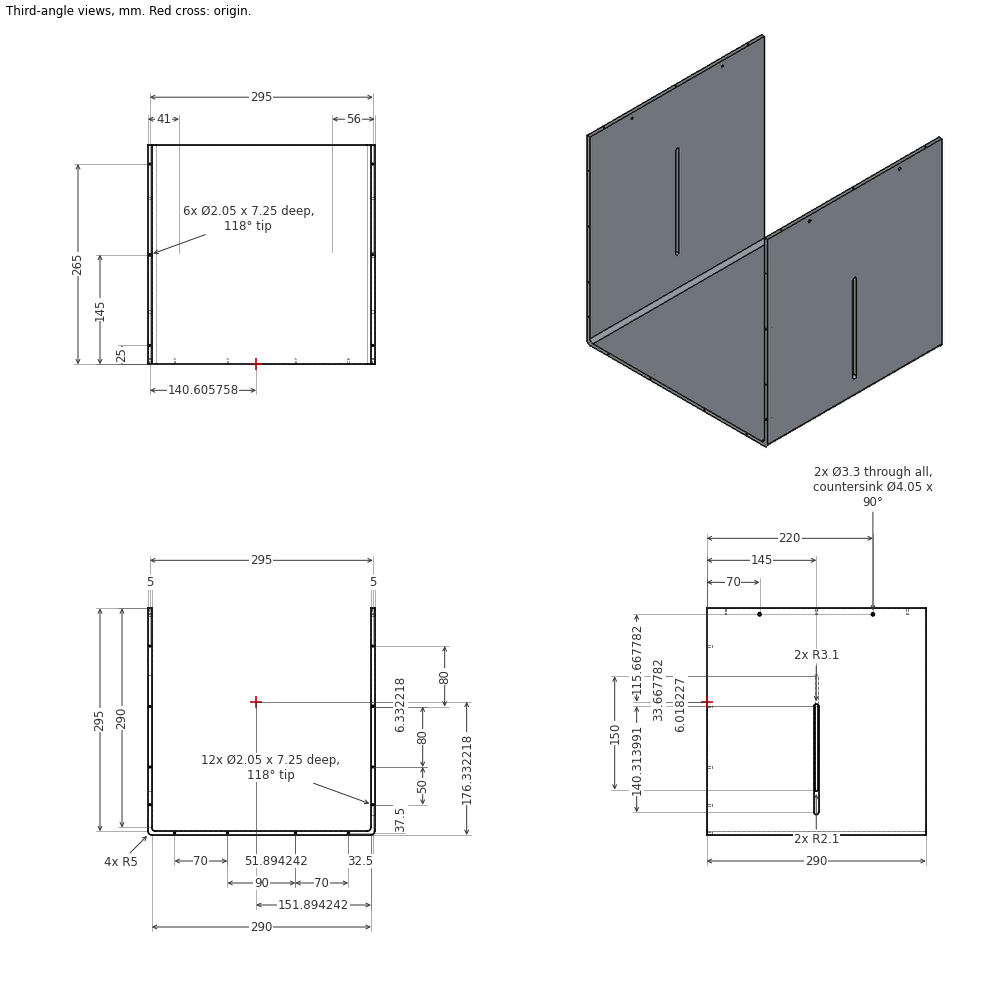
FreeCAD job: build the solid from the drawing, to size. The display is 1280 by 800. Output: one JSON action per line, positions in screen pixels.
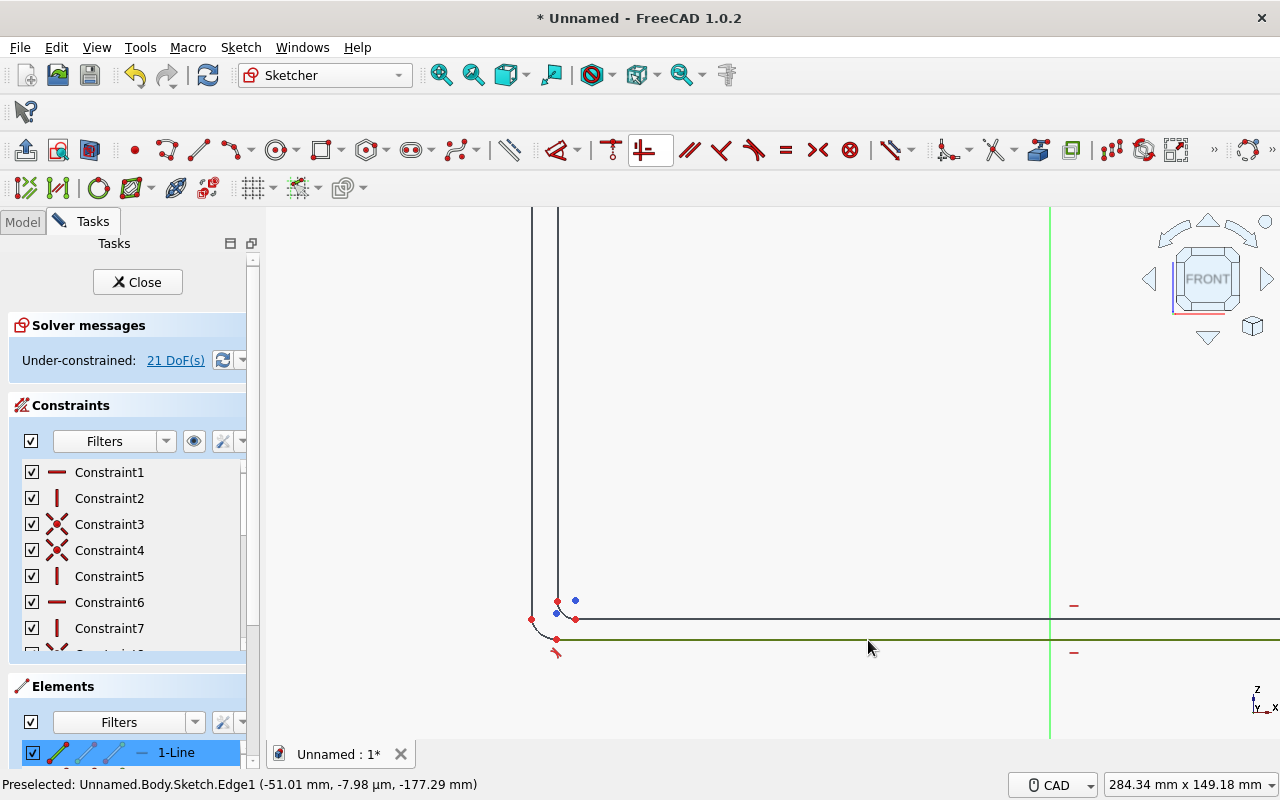
{"action": "scroll", "coordinate": [545, 633], "scroll_direction": "down", "scroll_amount": 6}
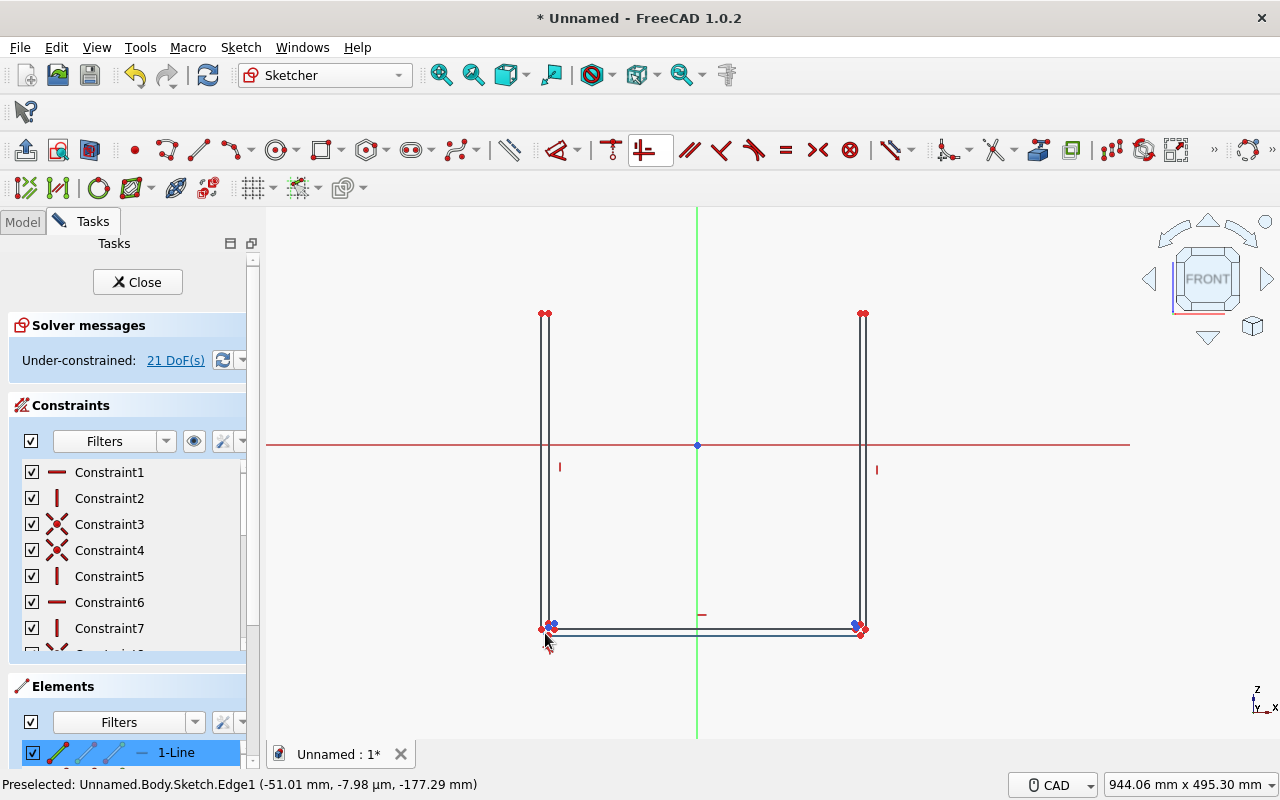
{"action": "scroll", "coordinate": [864, 633], "scroll_direction": "up", "scroll_amount": 7}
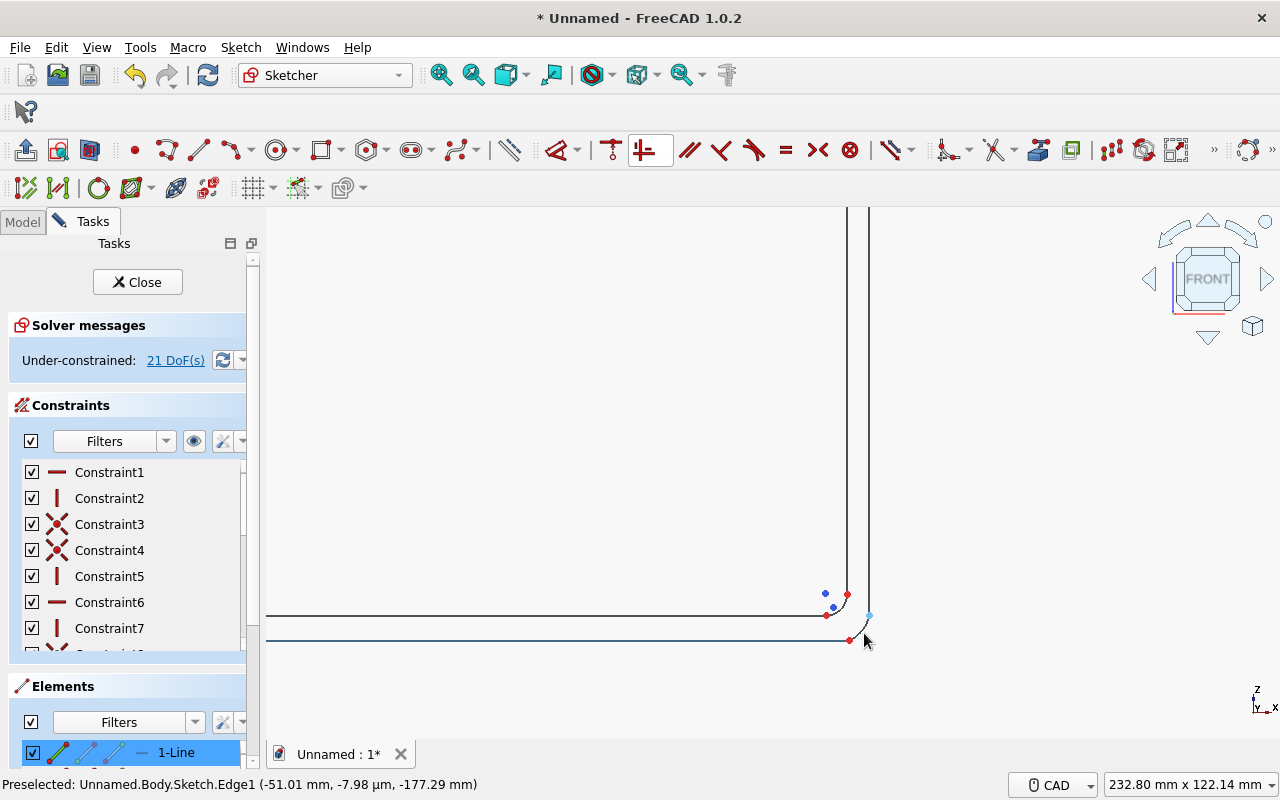
{"action": "left_click", "coordinate": [862, 631]}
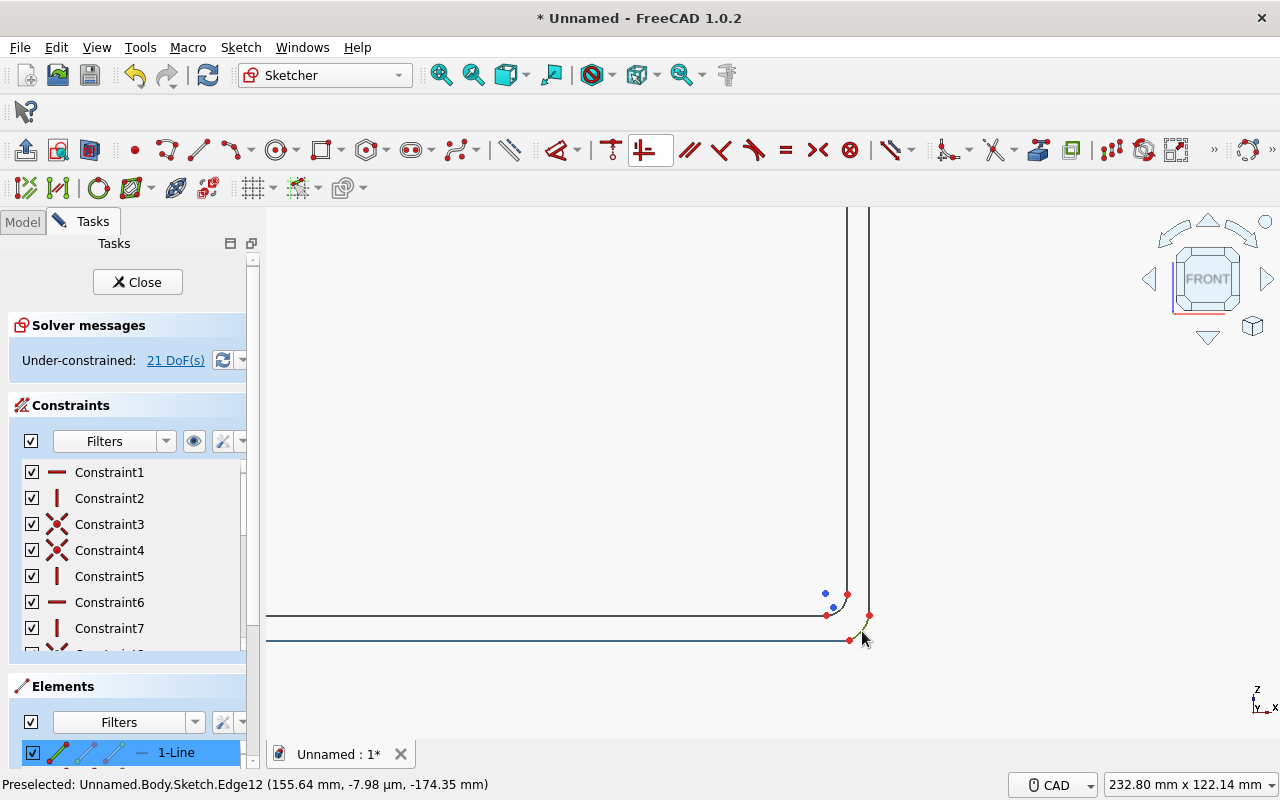
{"action": "left_click", "coordinate": [754, 150]}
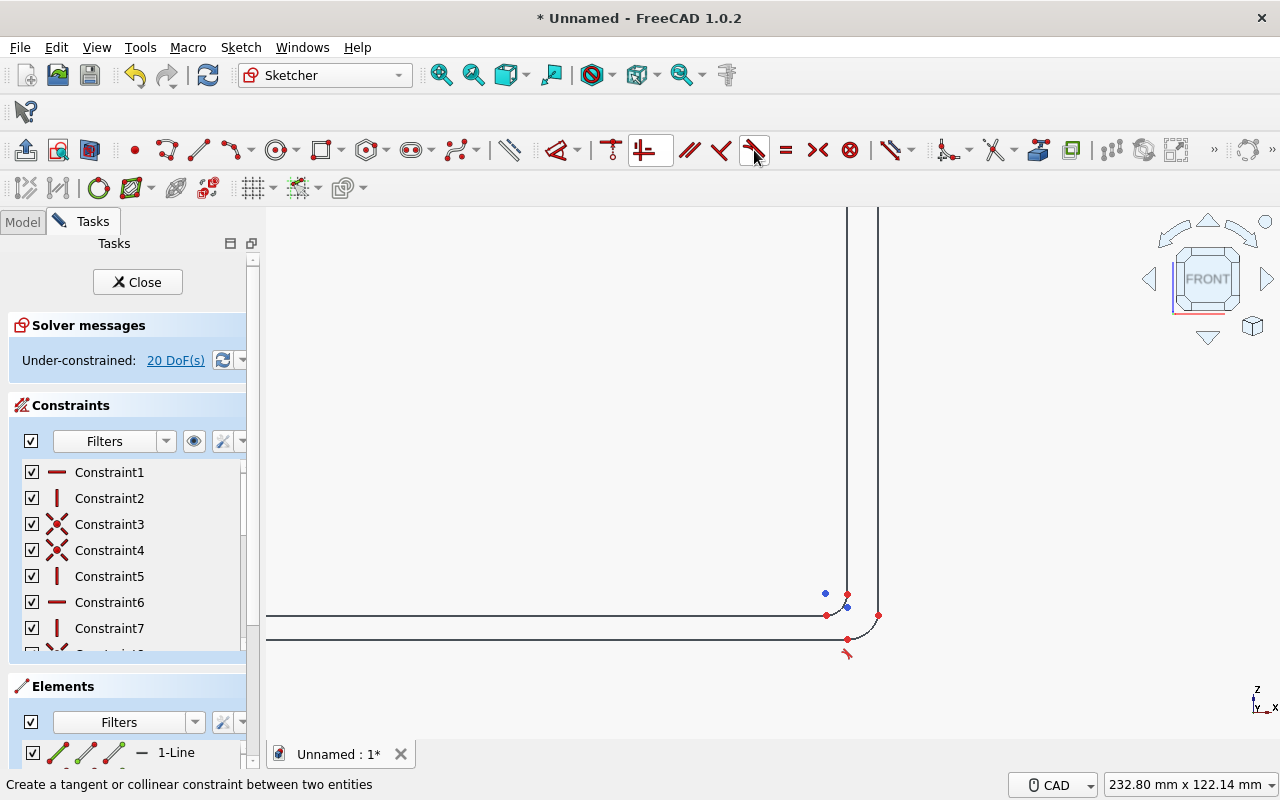
{"action": "scroll", "coordinate": [864, 633], "scroll_direction": "down", "scroll_amount": 7}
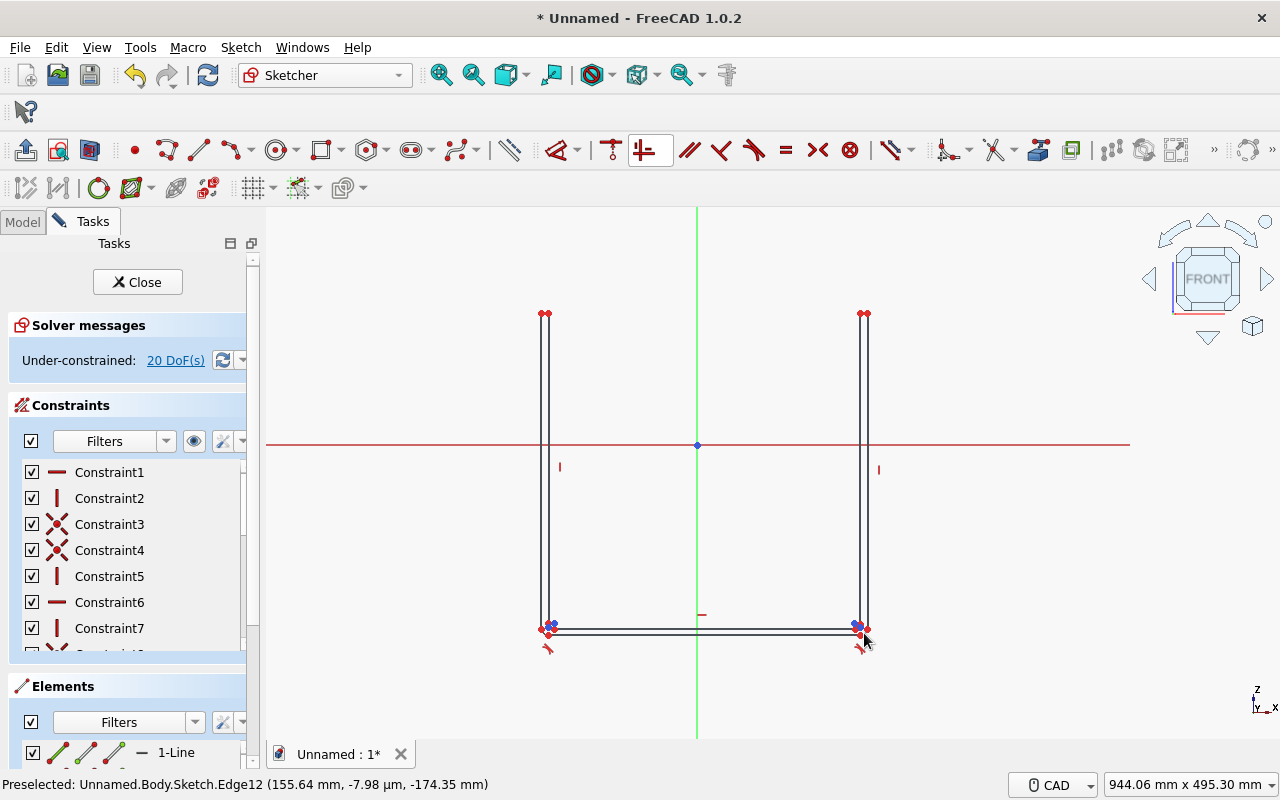
{"action": "scroll", "coordinate": [541, 535], "scroll_direction": "up", "scroll_amount": 4}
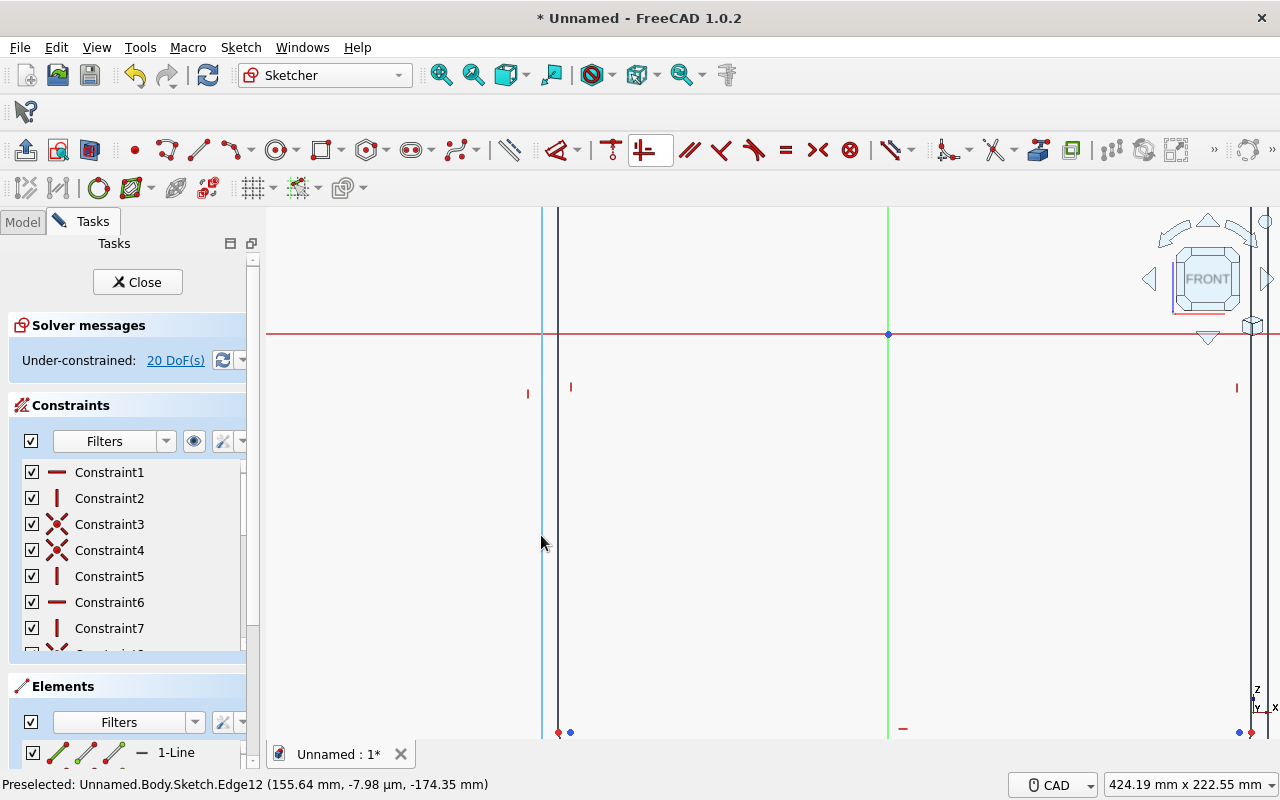
{"action": "left_click", "coordinate": [542, 534]}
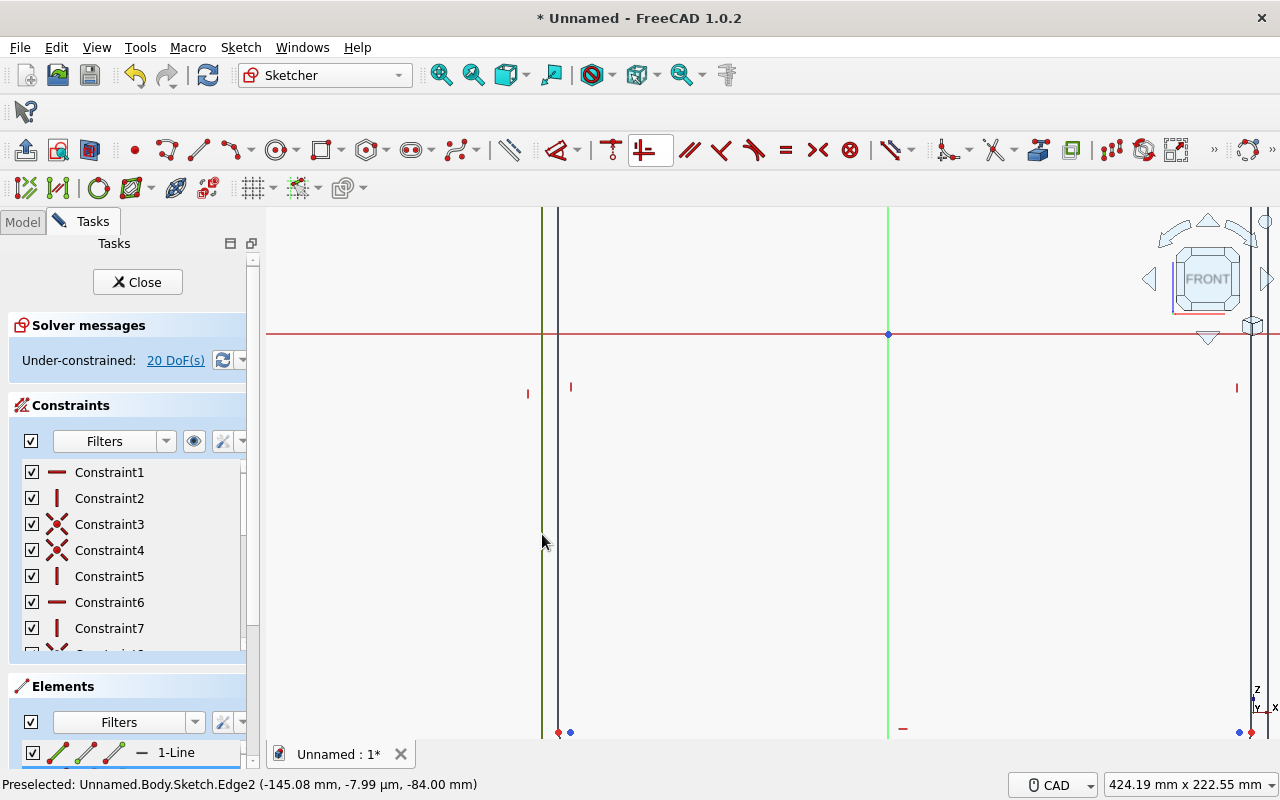
{"action": "scroll", "coordinate": [541, 535], "scroll_direction": "down", "scroll_amount": 4}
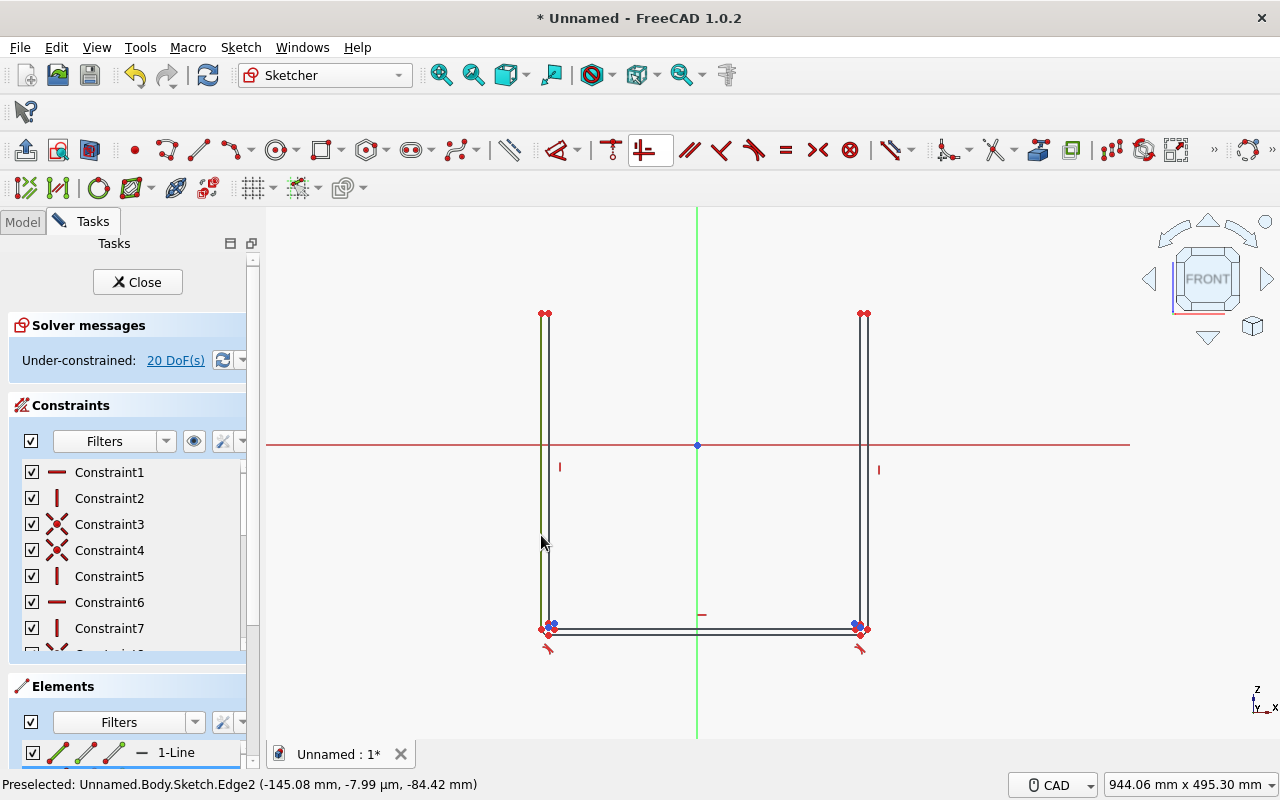
{"action": "scroll", "coordinate": [544, 634], "scroll_direction": "up", "scroll_amount": 6}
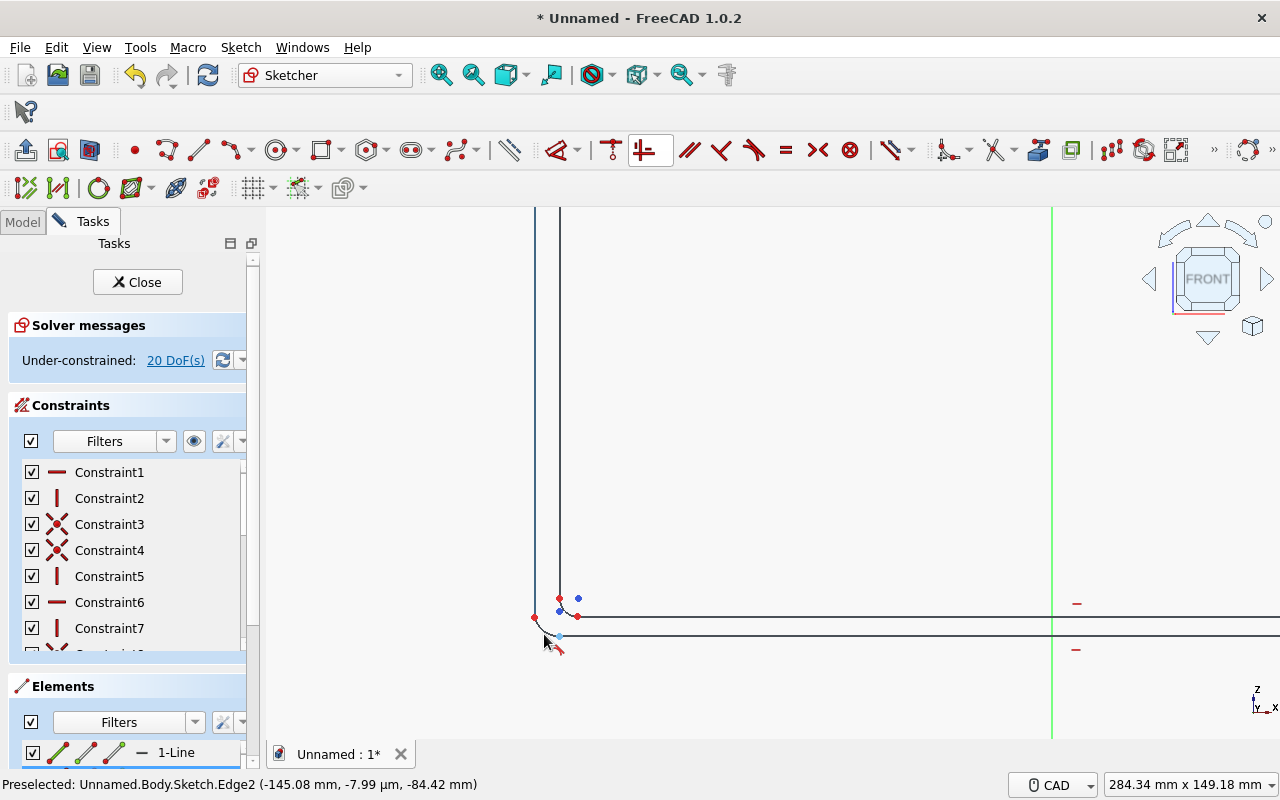
{"action": "left_click", "coordinate": [544, 631]}